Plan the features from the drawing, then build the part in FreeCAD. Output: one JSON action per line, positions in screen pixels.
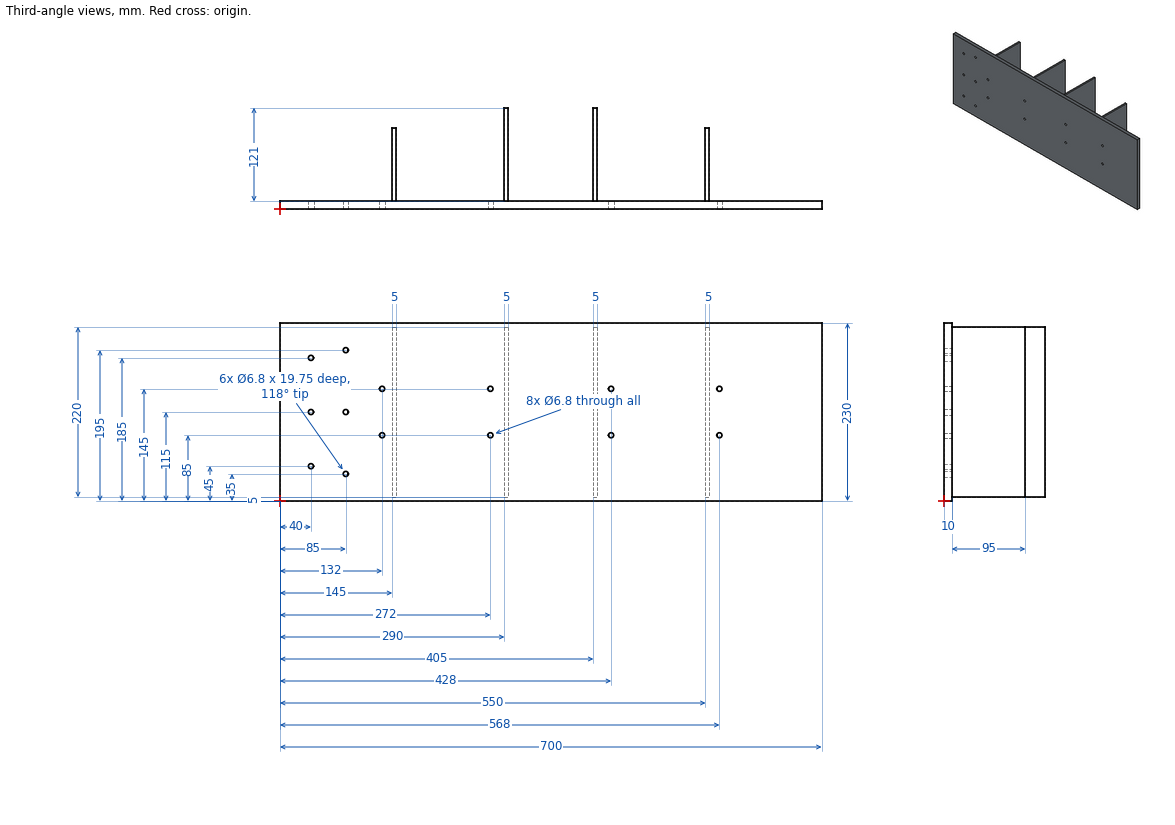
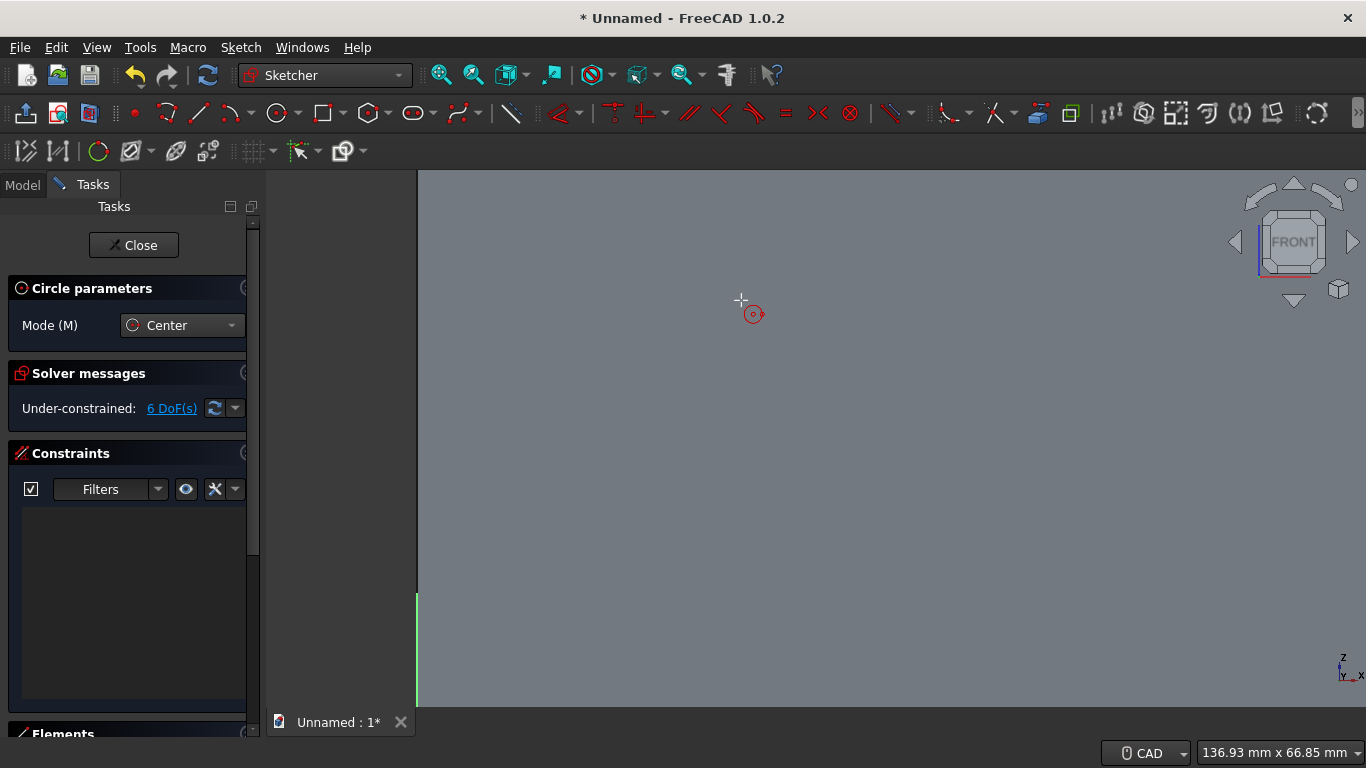
{"action": "scroll", "coordinate": [741, 299], "scroll_direction": "down", "scroll_amount": 8}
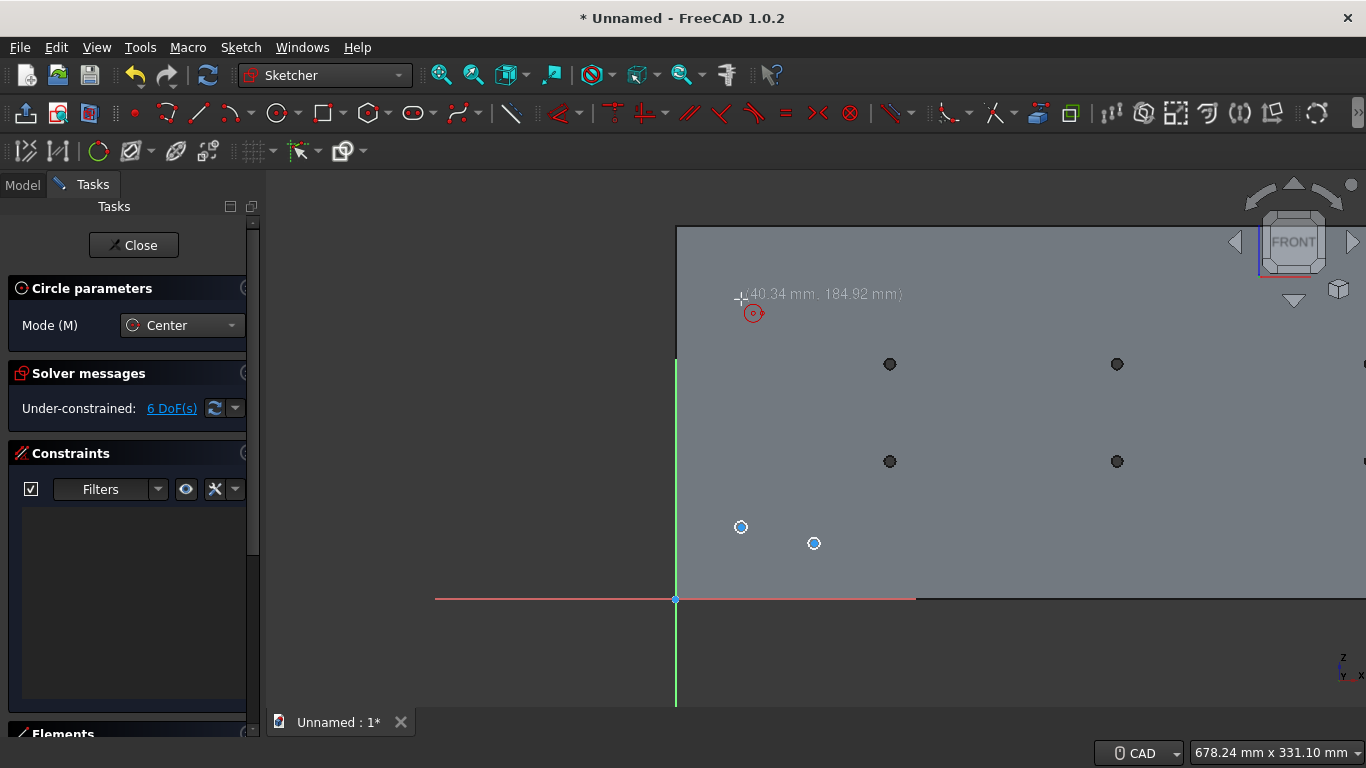
{"action": "left_click", "coordinate": [741, 299]}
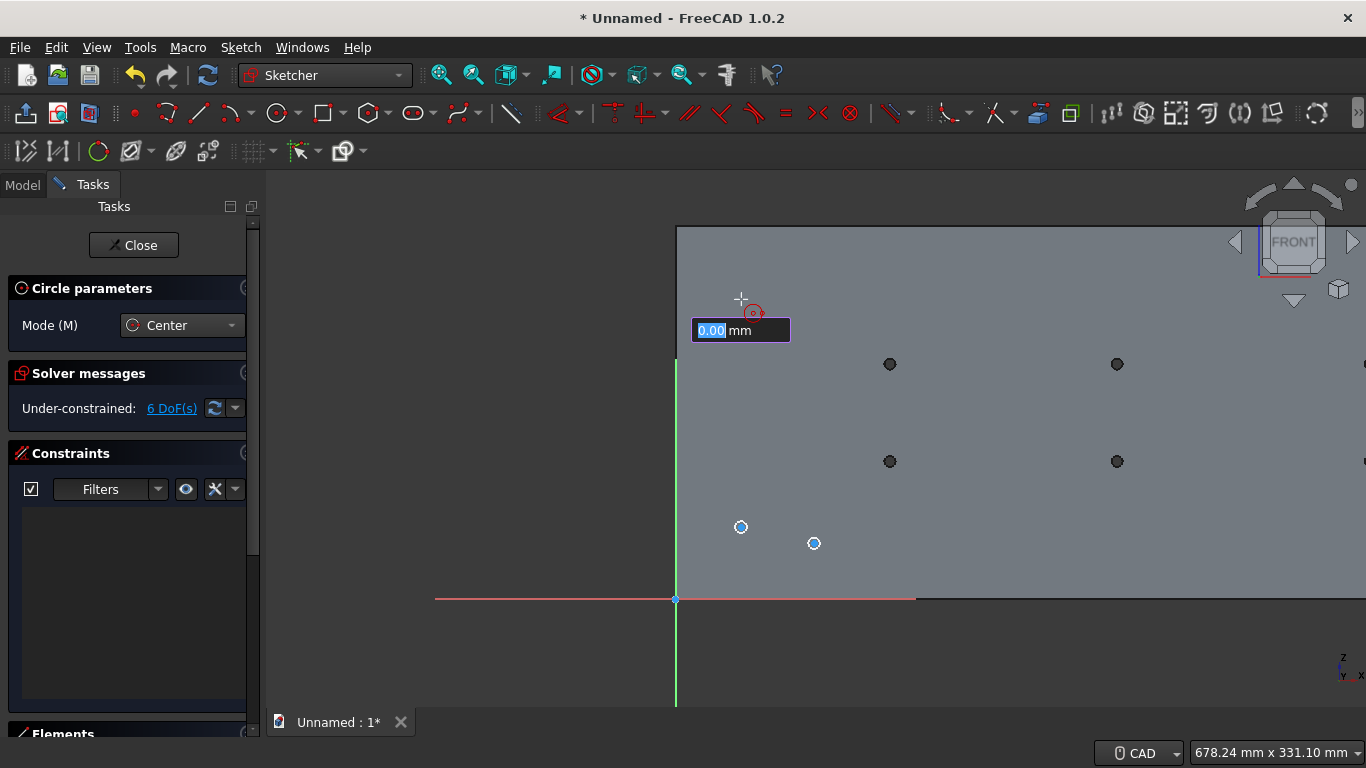
{"action": "scroll", "coordinate": [745, 295], "scroll_direction": "up", "scroll_amount": 6}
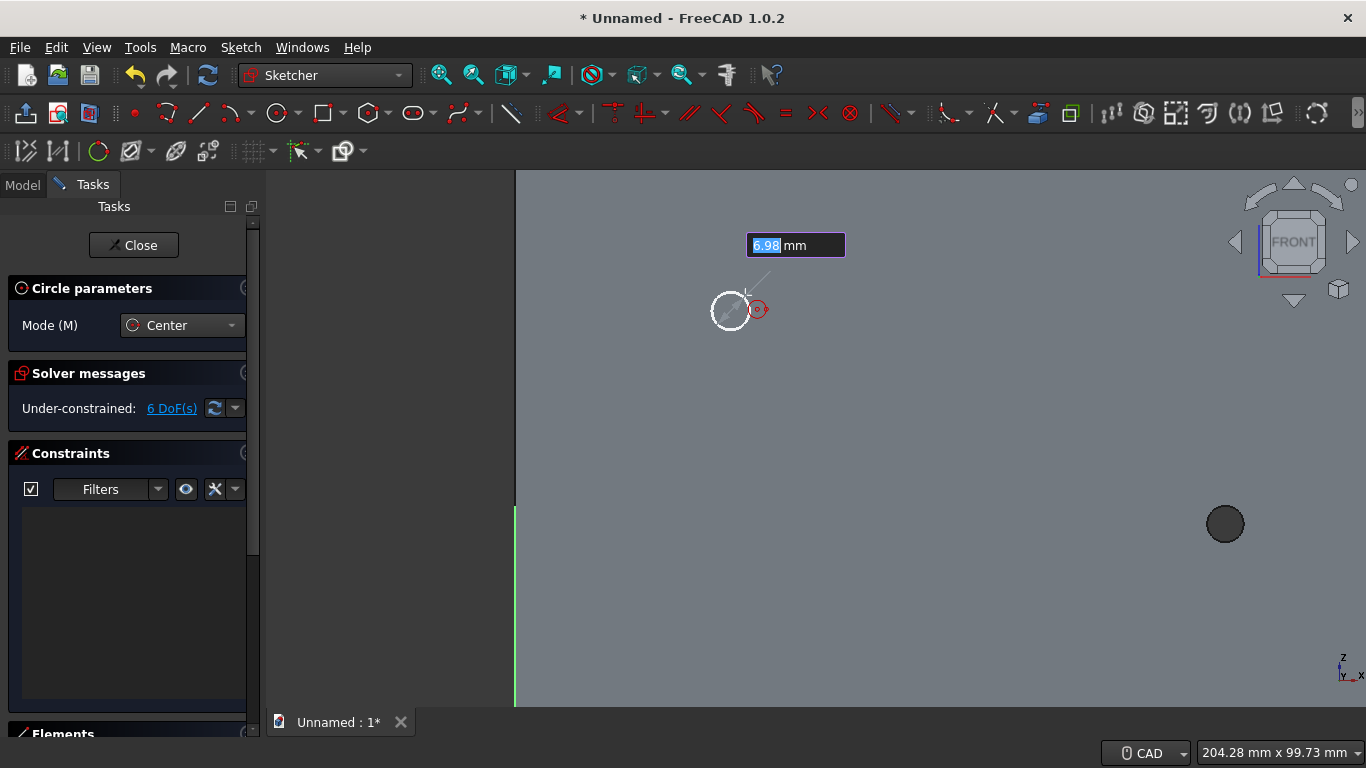
{"action": "left_click", "coordinate": [743, 296]}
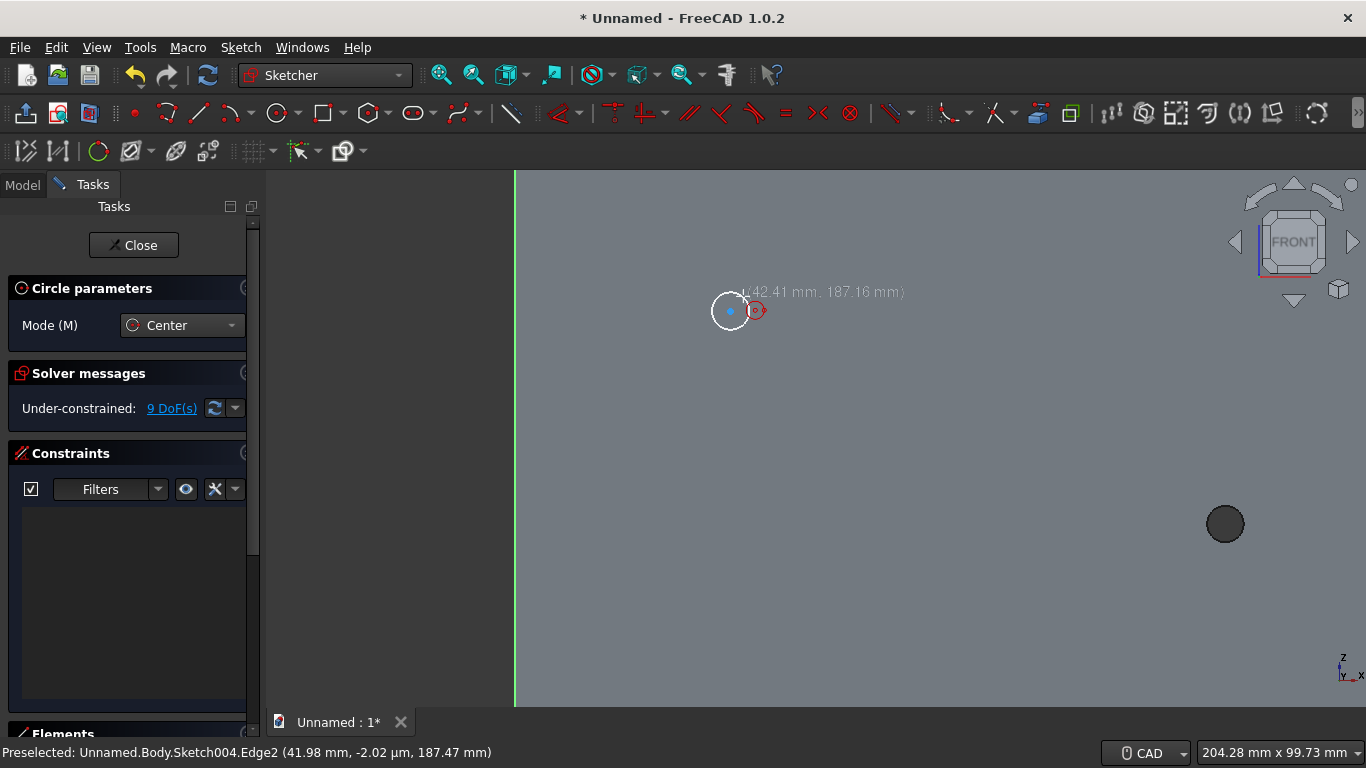
{"action": "scroll", "coordinate": [972, 255], "scroll_direction": "up", "scroll_amount": 2}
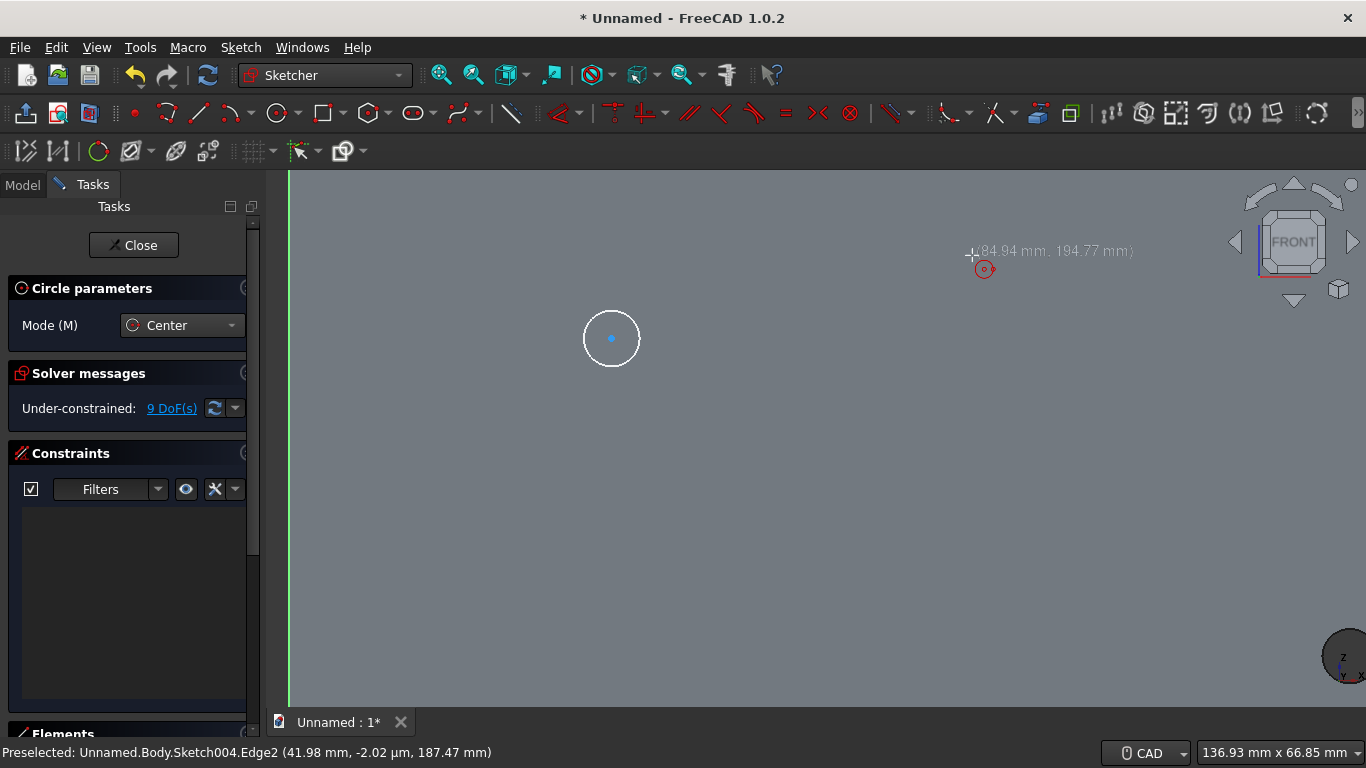
{"action": "scroll", "coordinate": [774, 290], "scroll_direction": "down", "scroll_amount": 8}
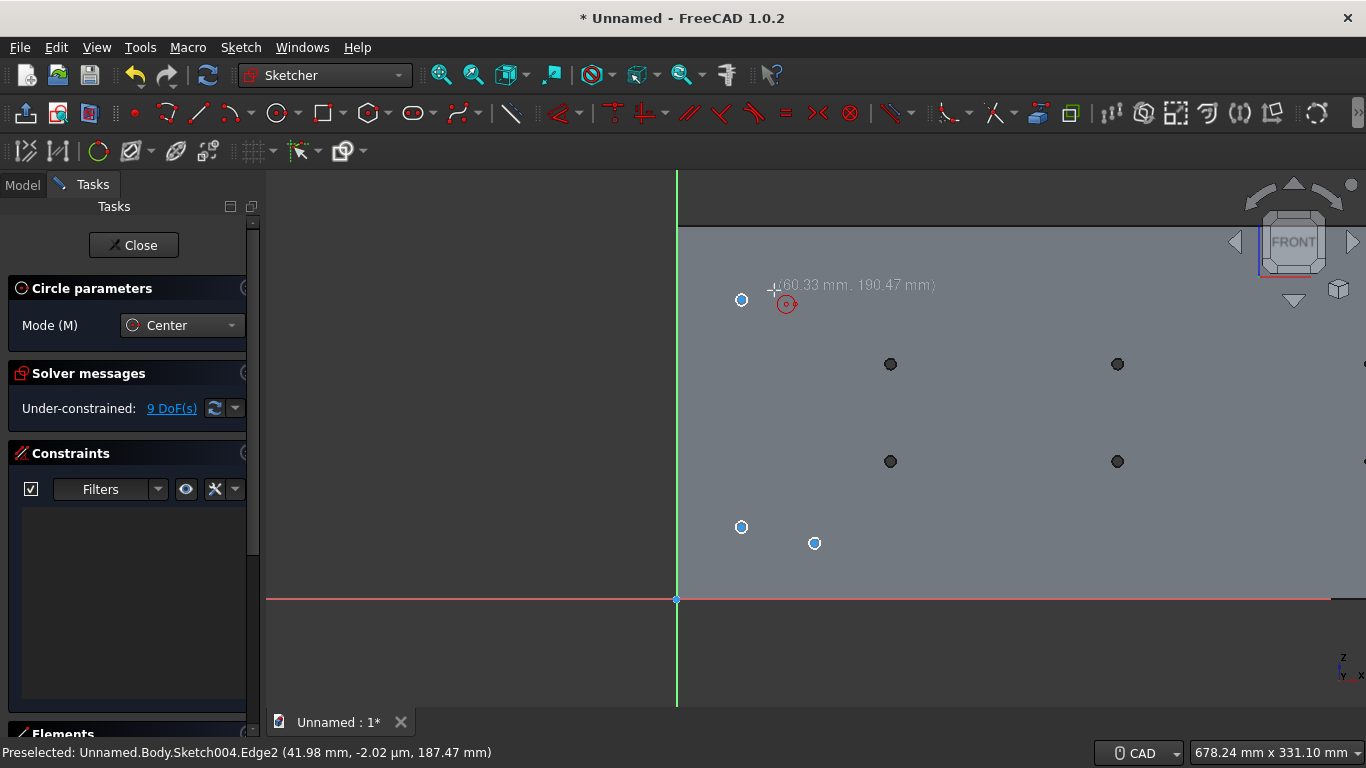
{"action": "left_click", "coordinate": [814, 283]}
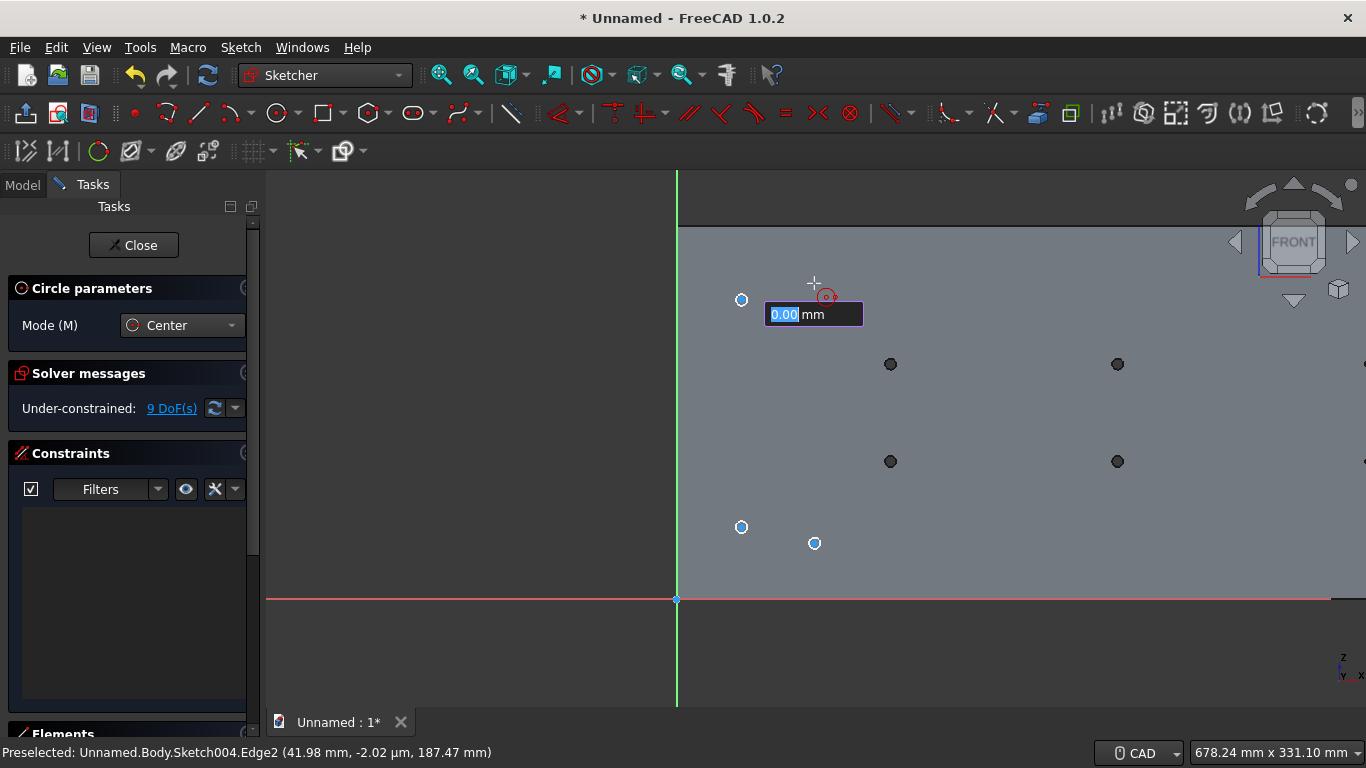
{"action": "scroll", "coordinate": [818, 279], "scroll_direction": "up", "scroll_amount": 6}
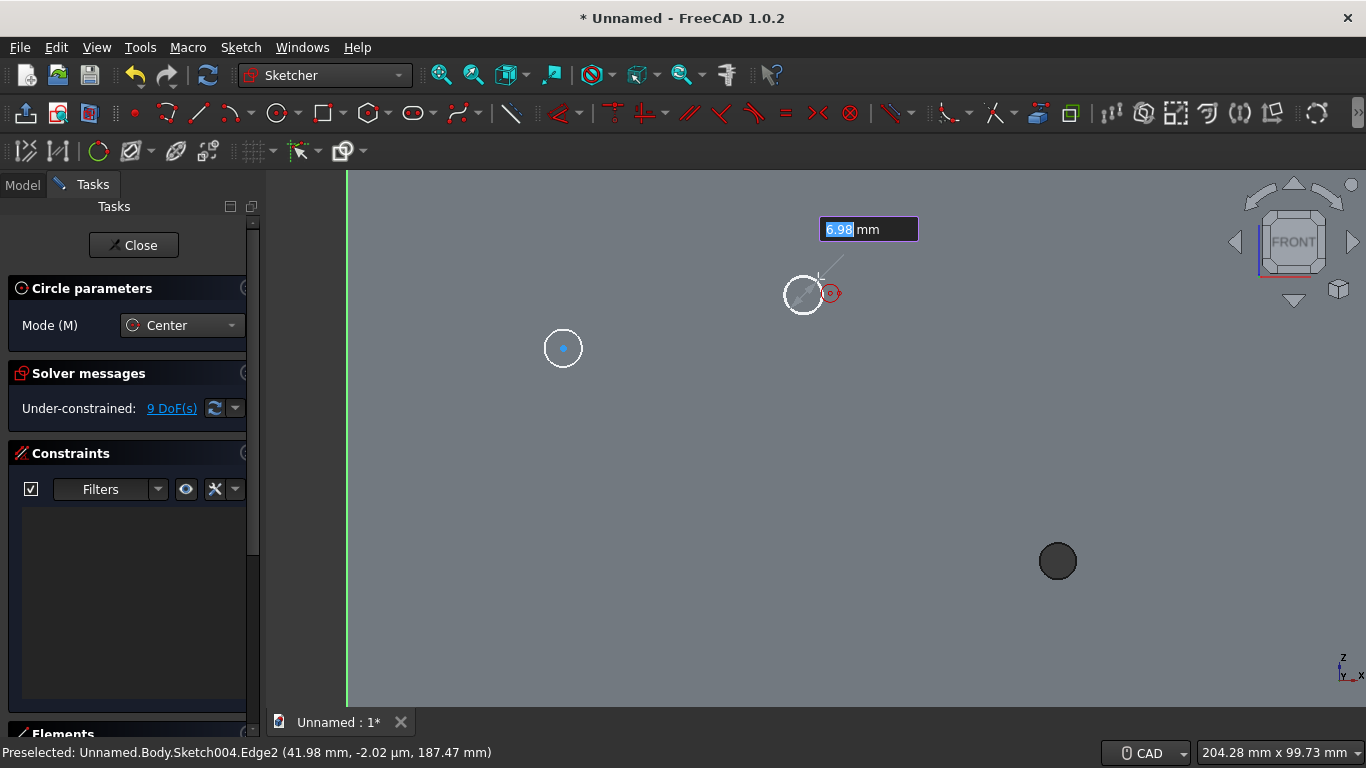
{"action": "left_click", "coordinate": [818, 279]}